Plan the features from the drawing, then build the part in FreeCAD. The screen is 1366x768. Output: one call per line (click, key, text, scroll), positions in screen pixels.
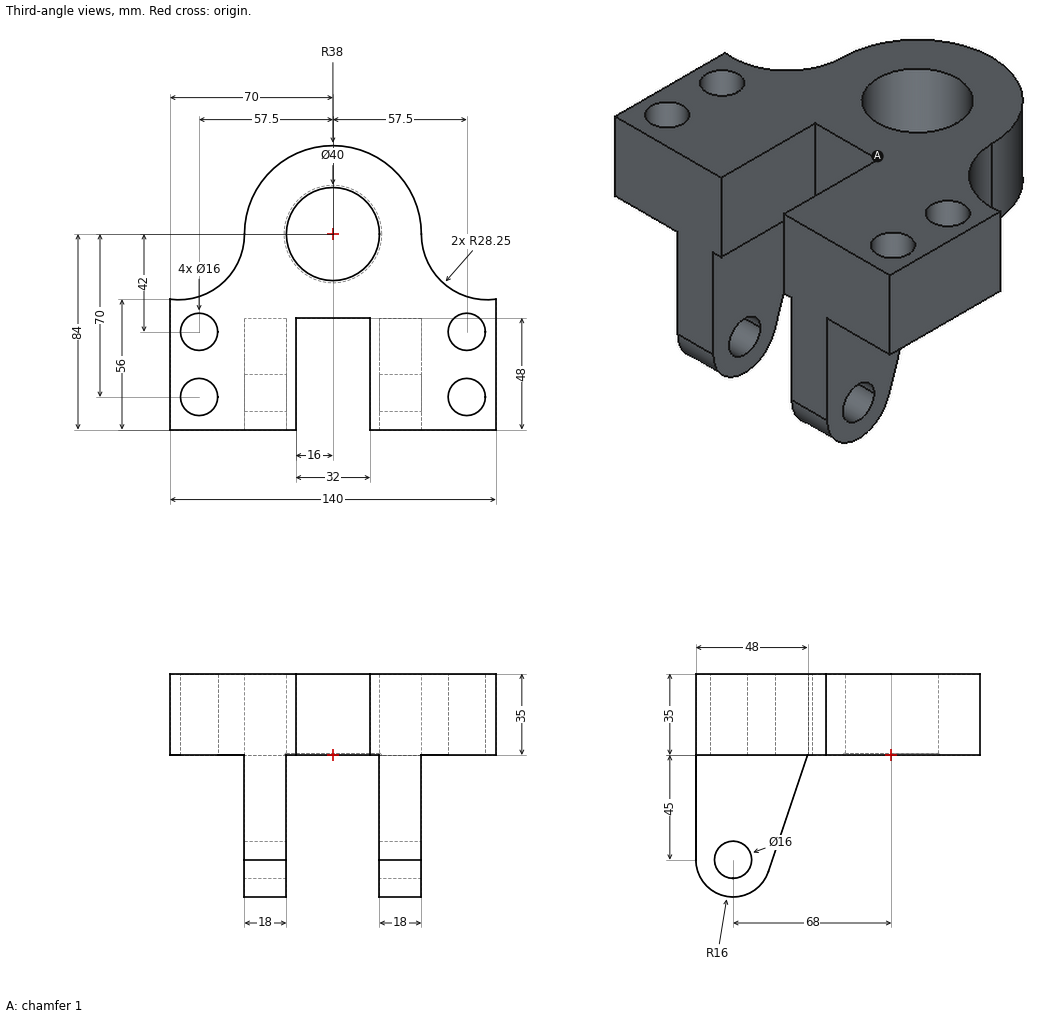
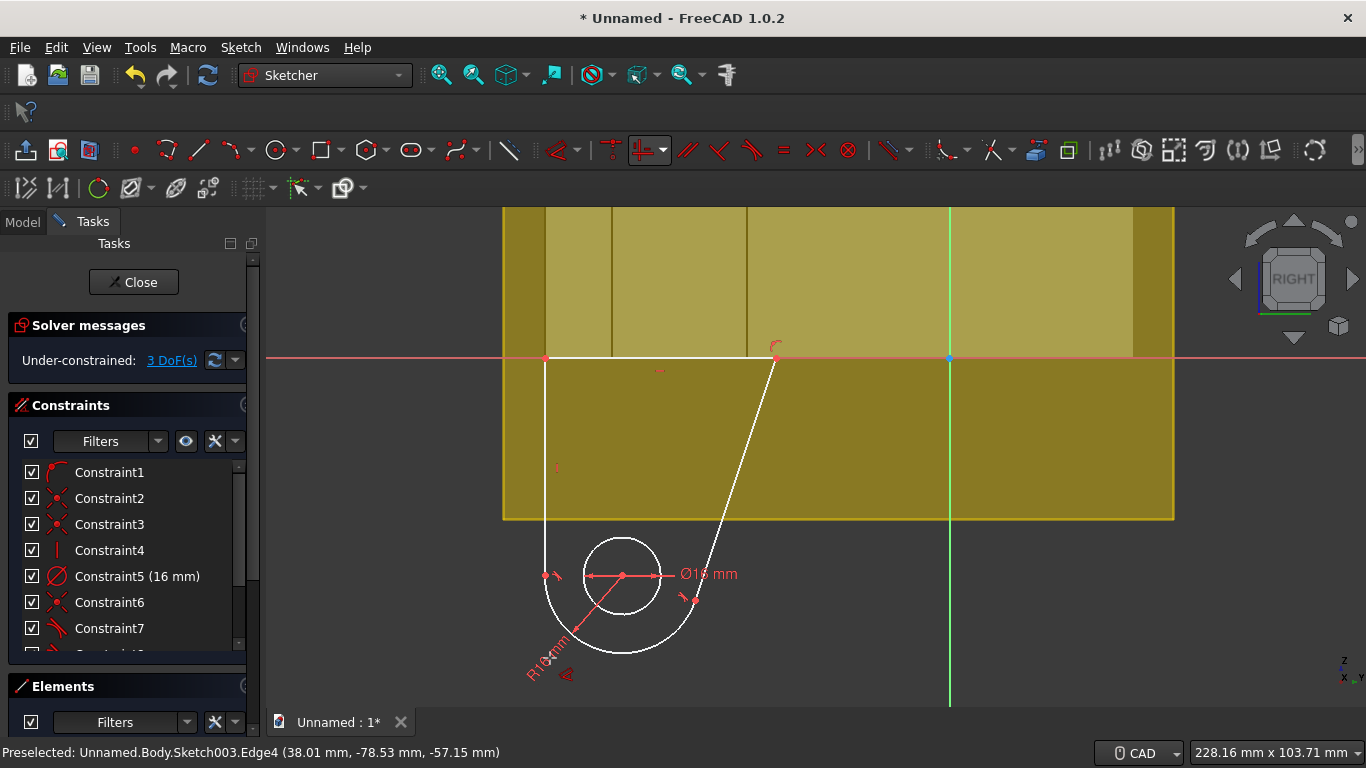
click(707, 358)
click(661, 324)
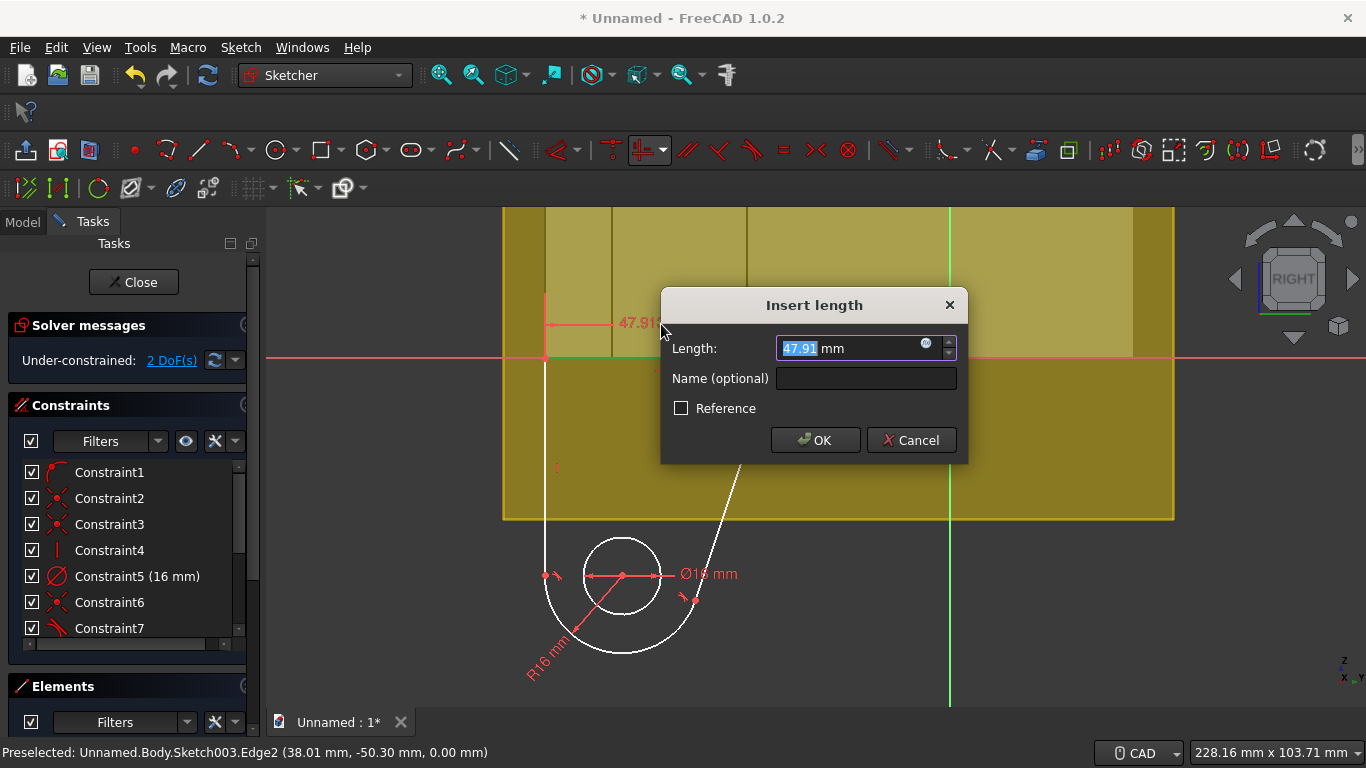
text(48)
key(Return)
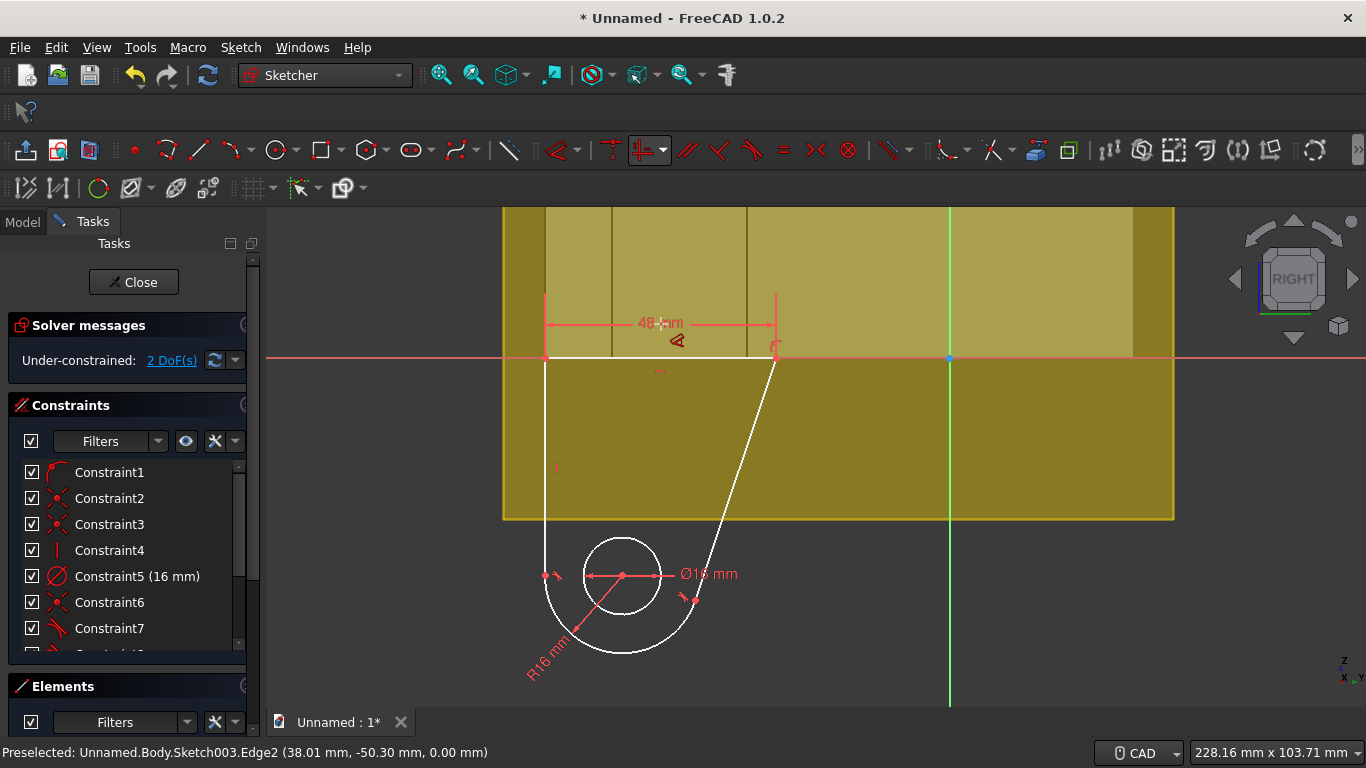
click(545, 423)
click(511, 467)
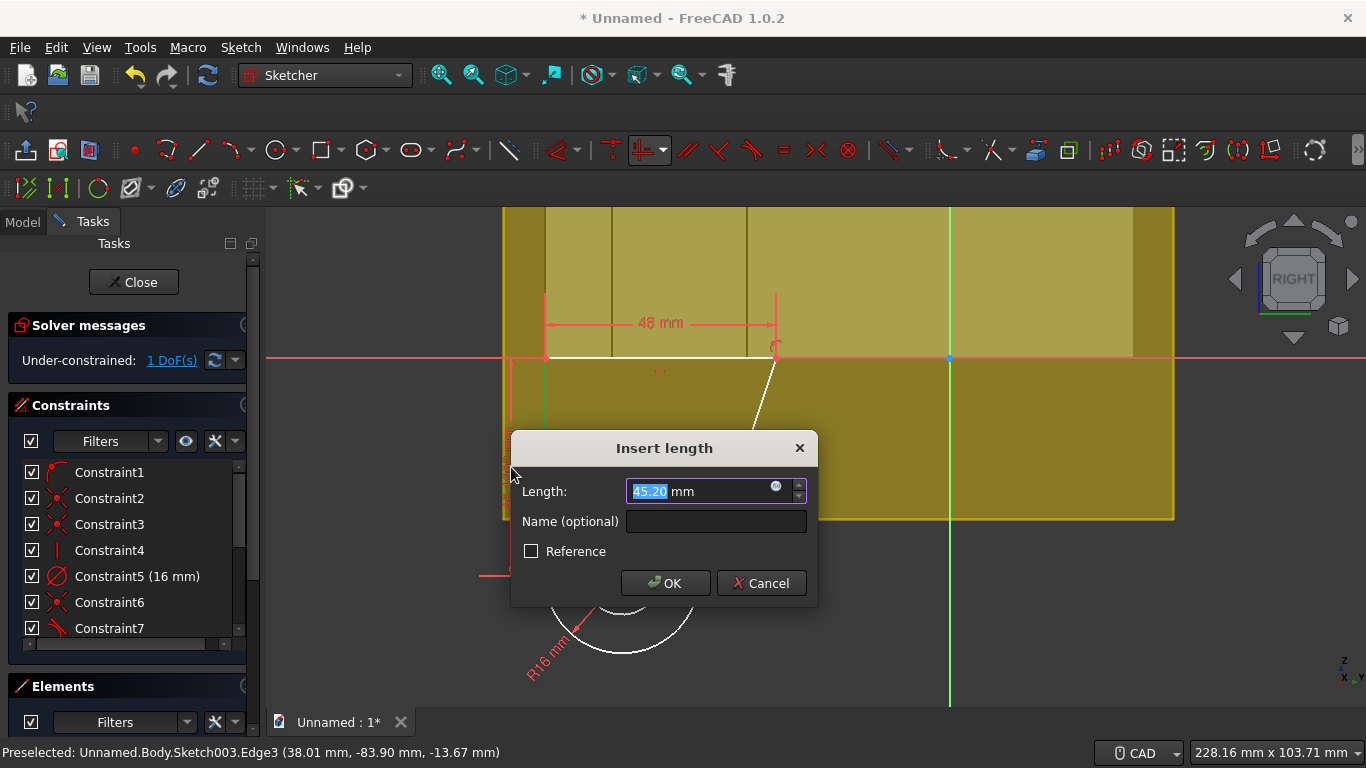
text(45)
key(Return)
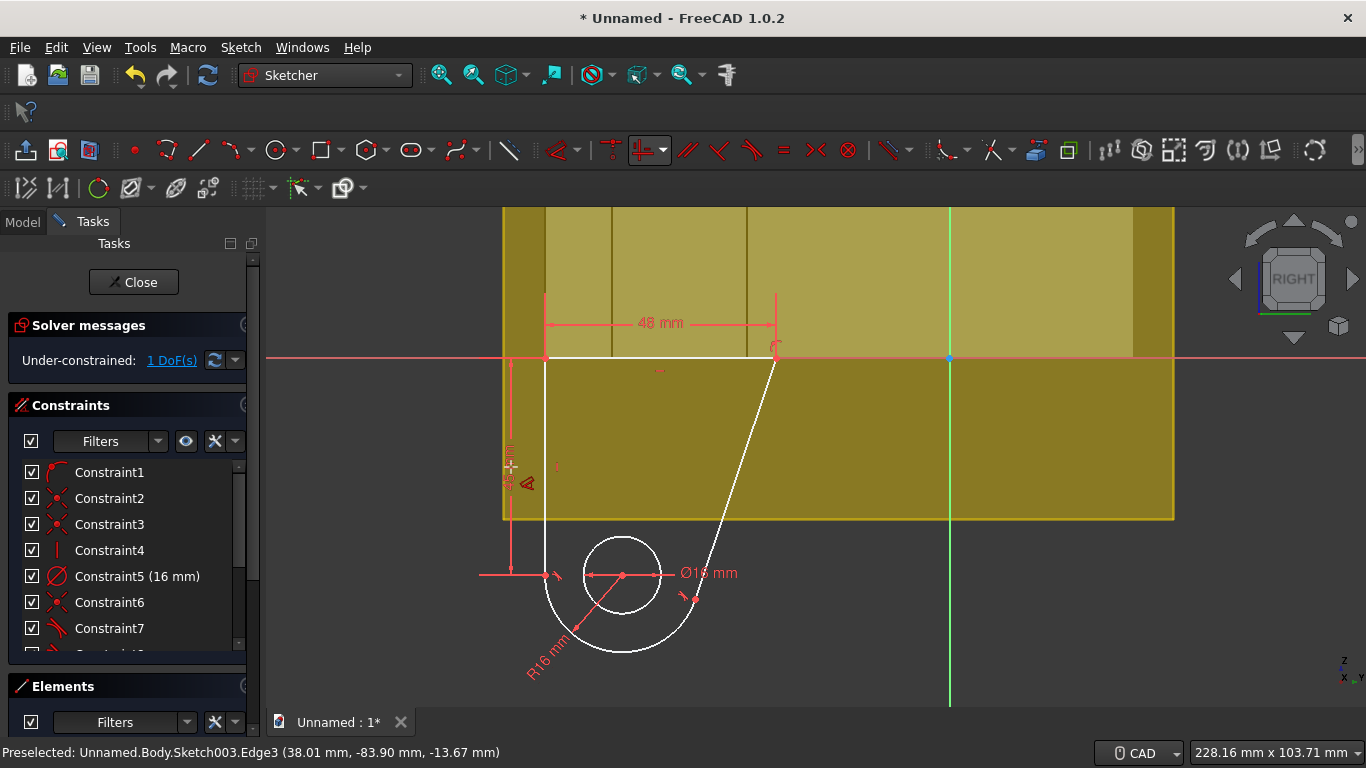
click(622, 575)
click(786, 324)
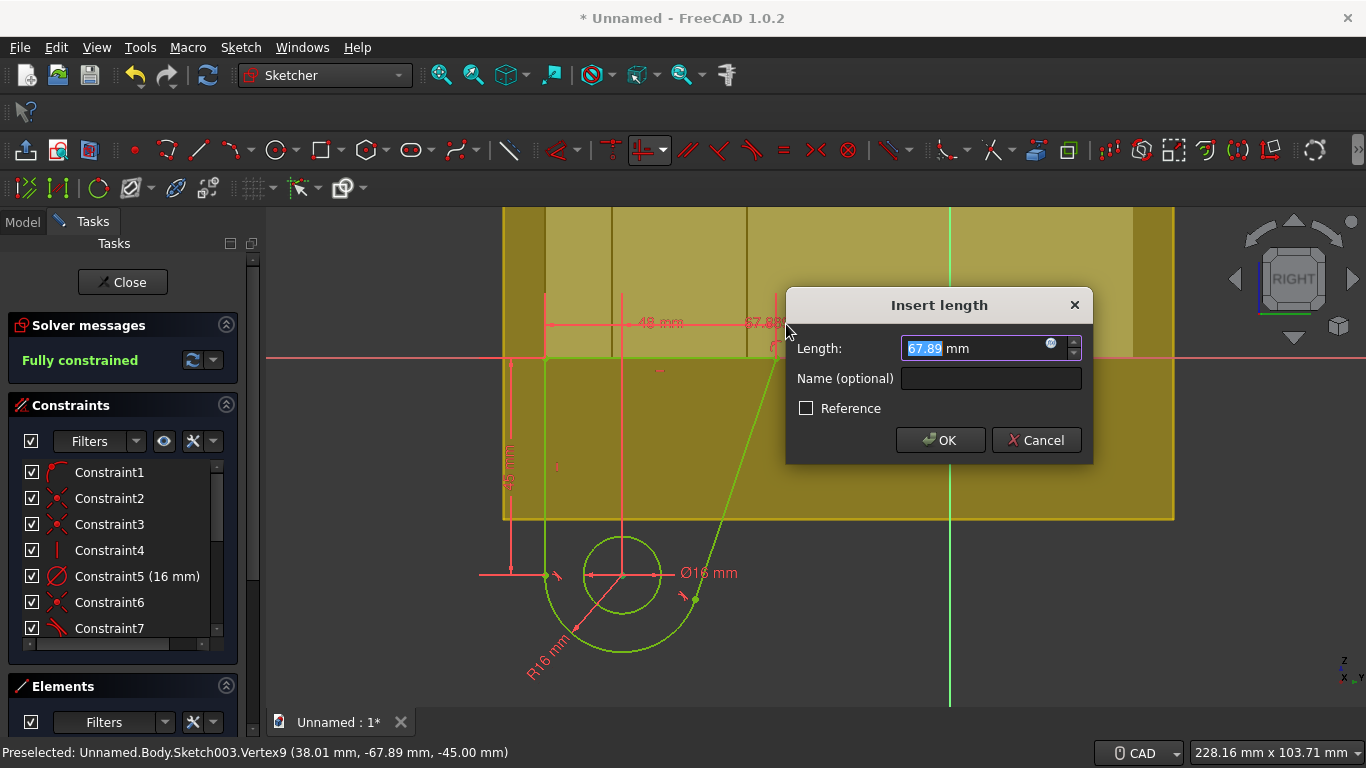
text(68)
key(Return)
key(Escape)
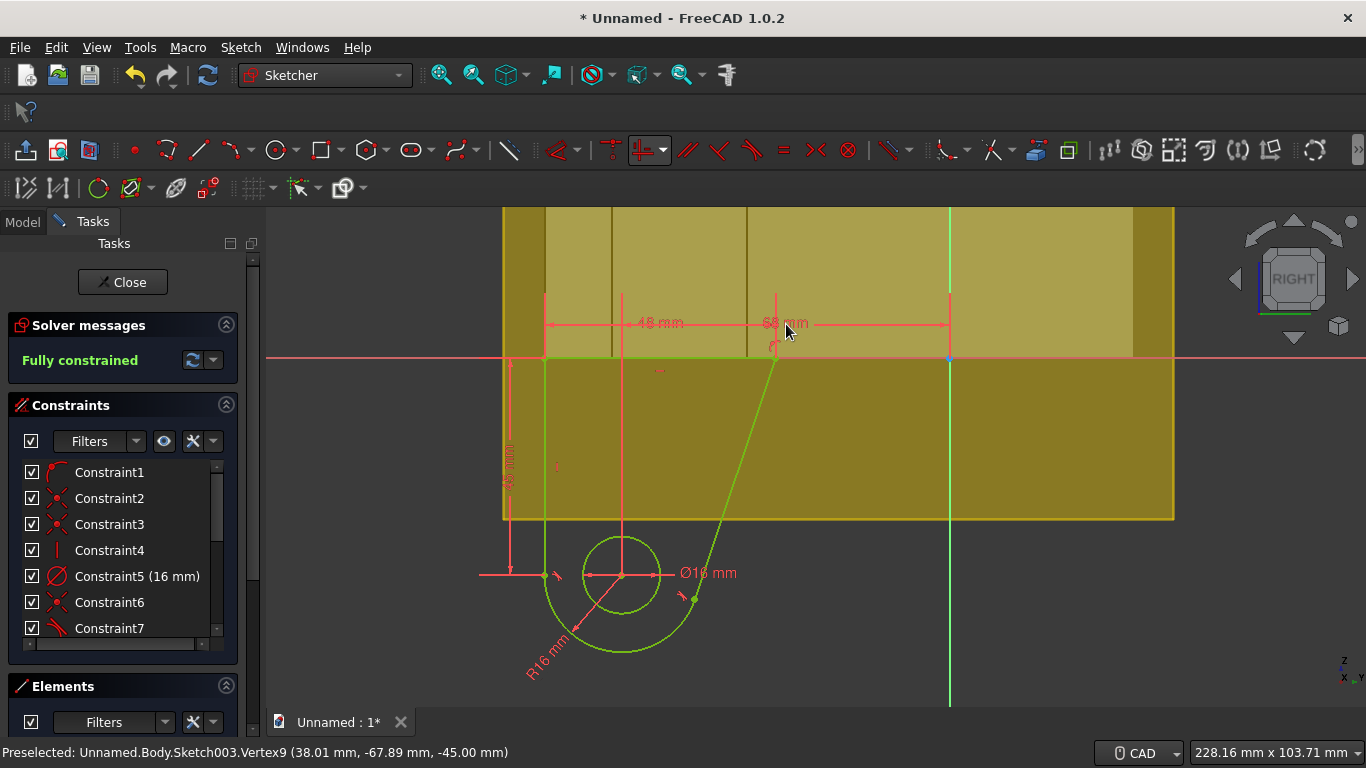
click(123, 282)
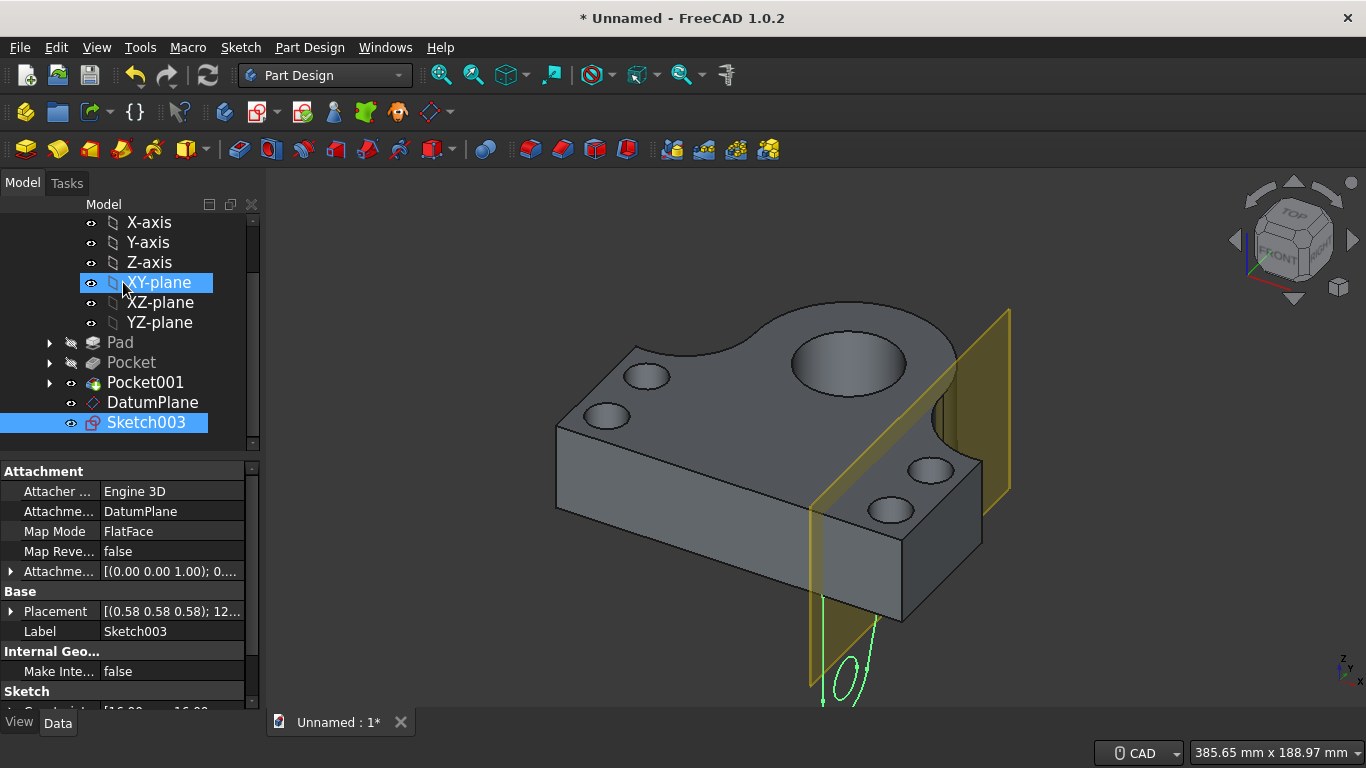
click(26, 150)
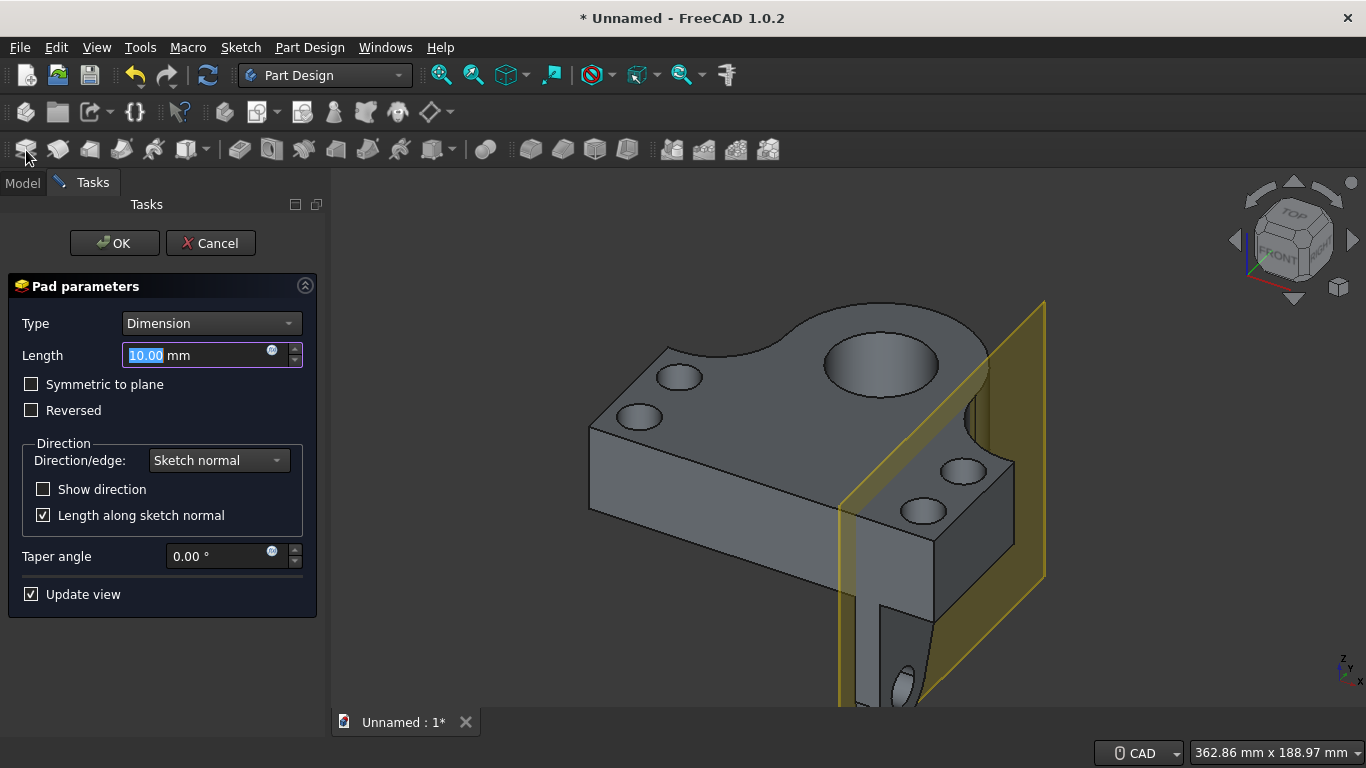
text(18)
key(Tab)